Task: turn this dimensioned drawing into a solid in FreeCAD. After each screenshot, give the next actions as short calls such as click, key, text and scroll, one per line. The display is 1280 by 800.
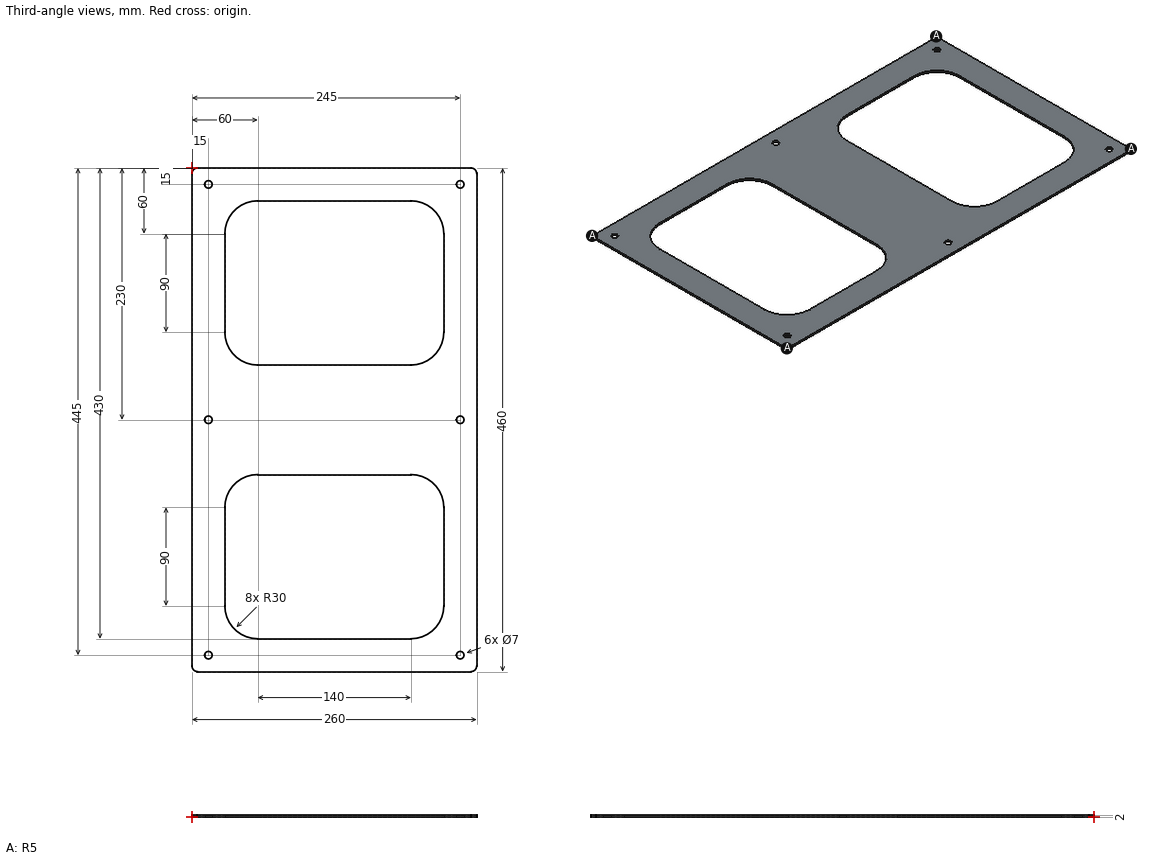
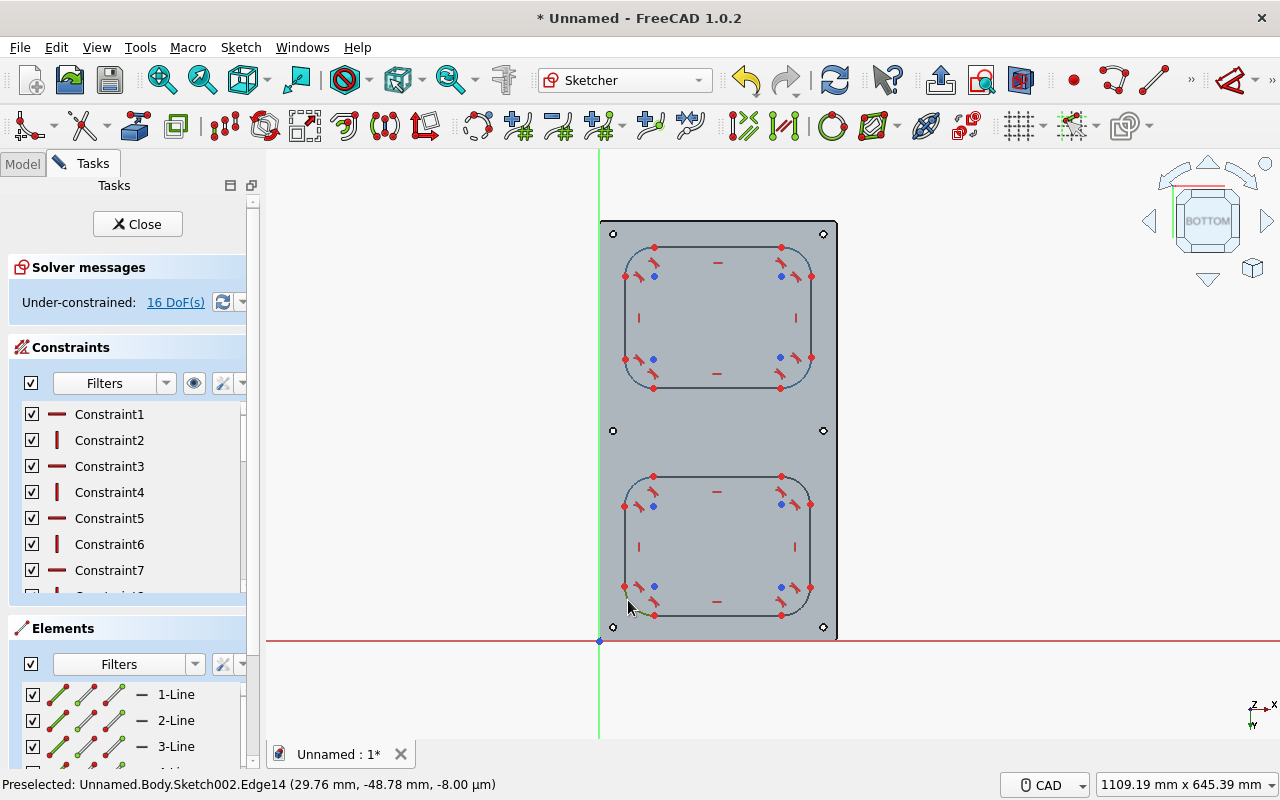
click(794, 613)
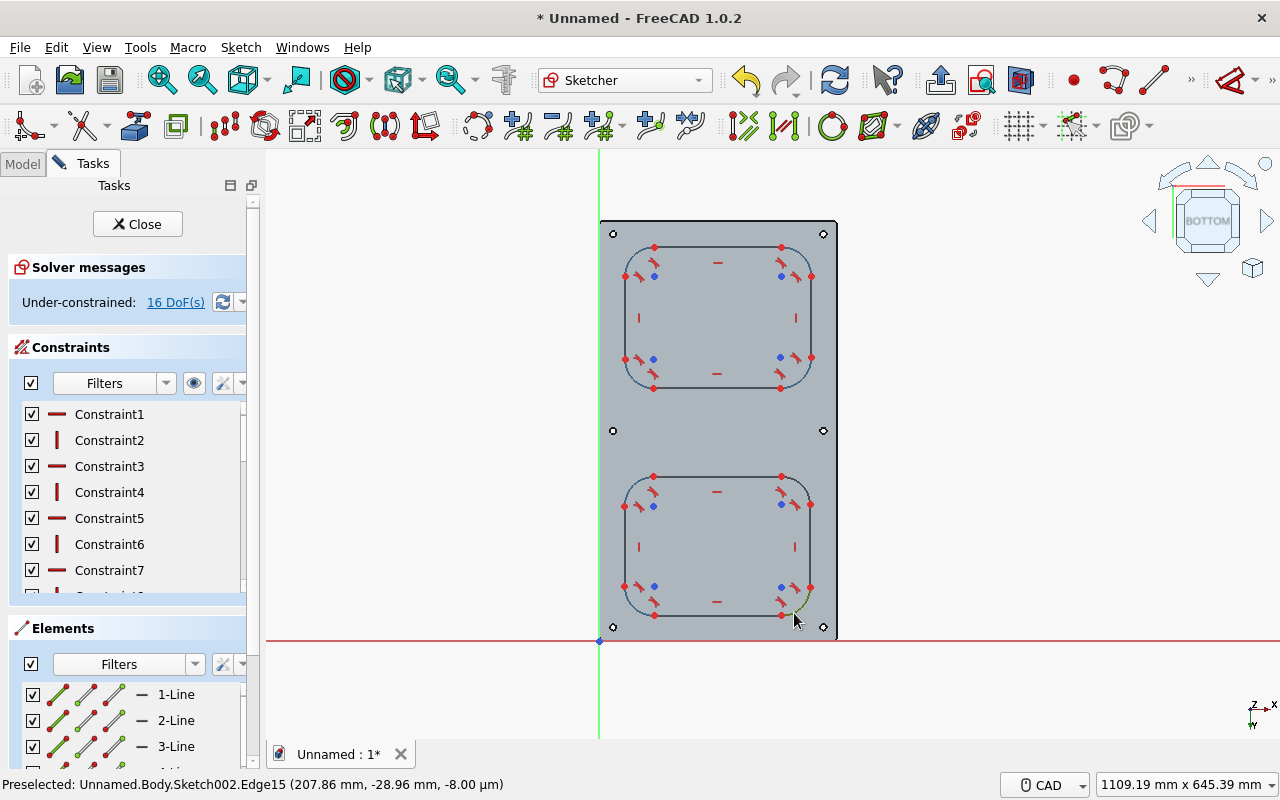
click(807, 492)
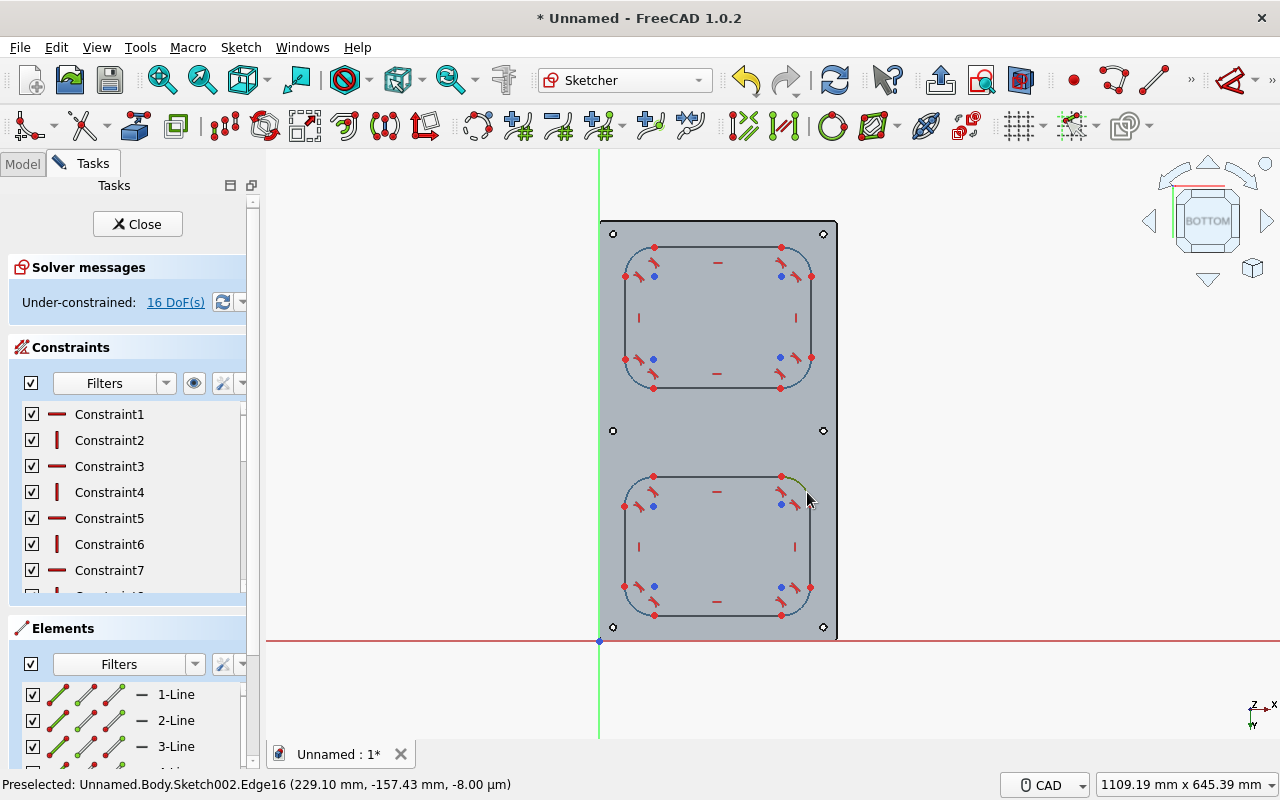
key(e)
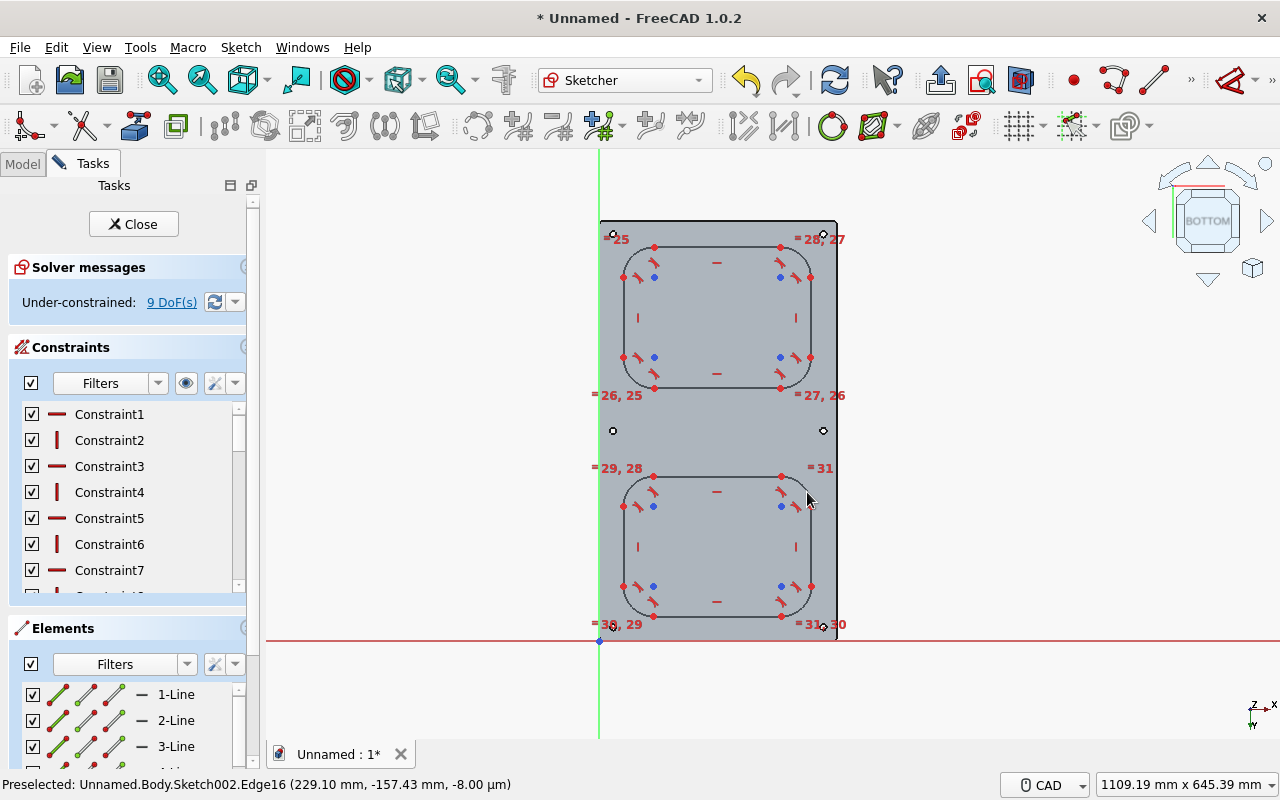
click(1230, 80)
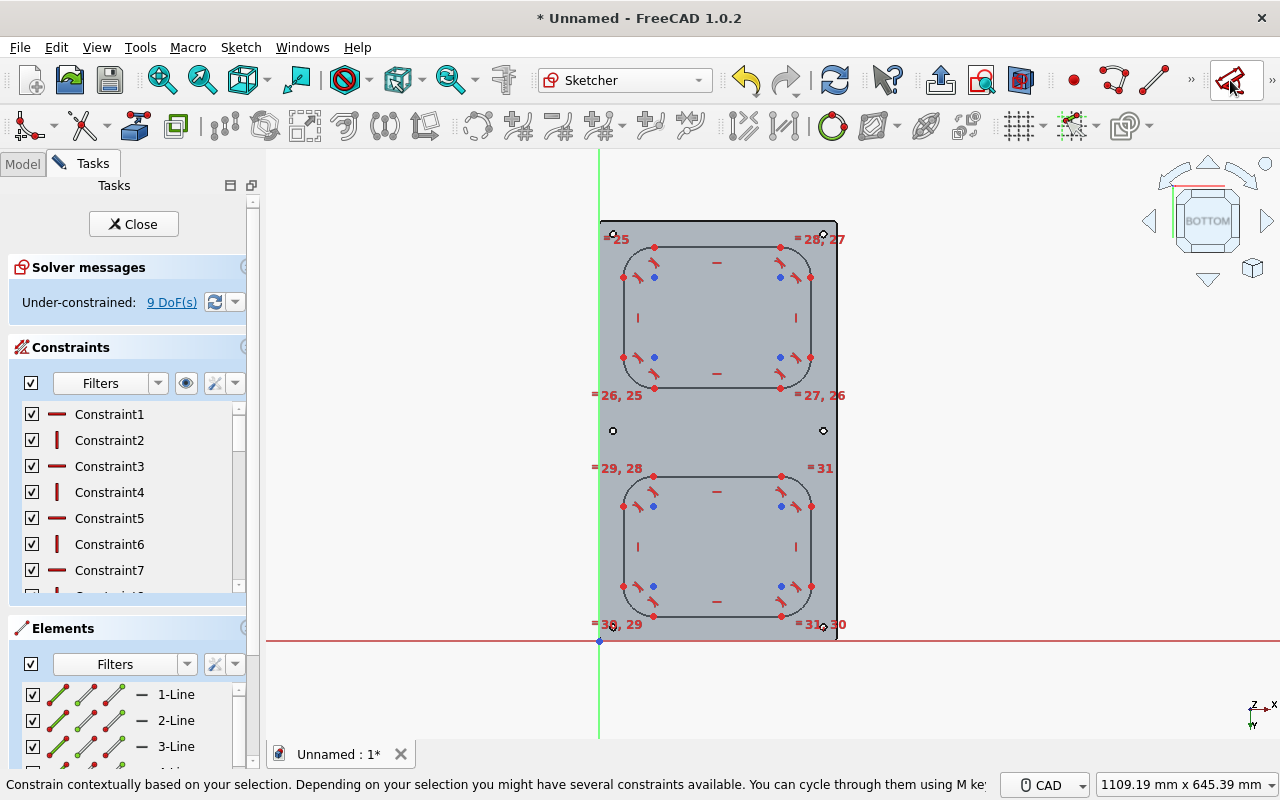
scroll(640, 251, up, 2)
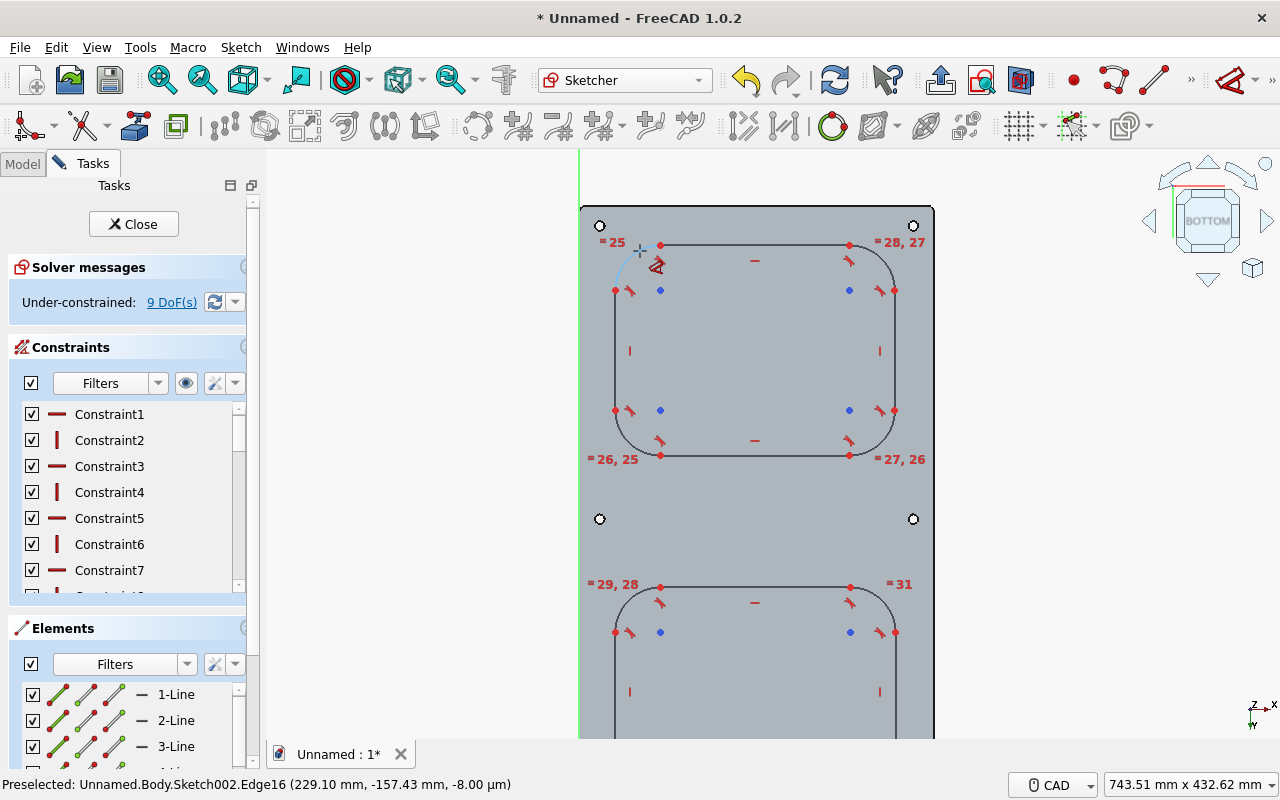
click(640, 250)
click(626, 221)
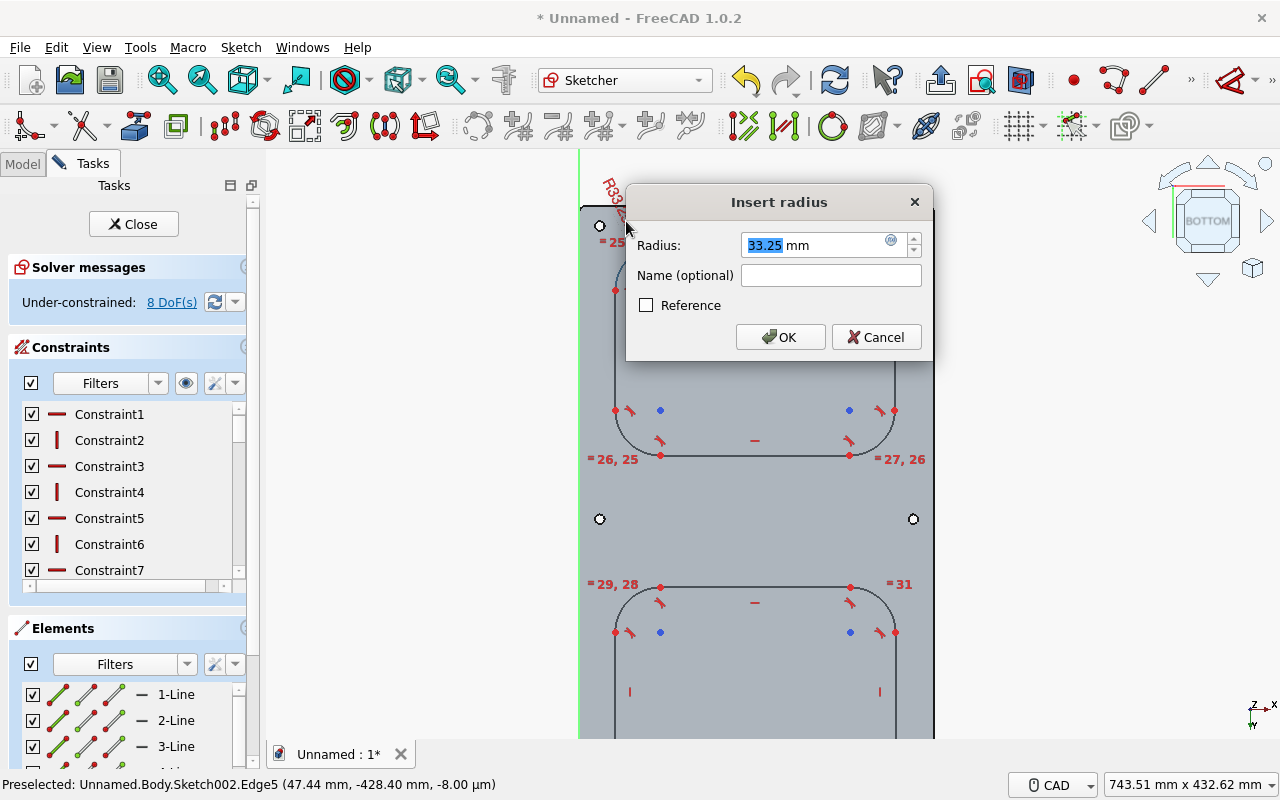
text(30)
key(Return)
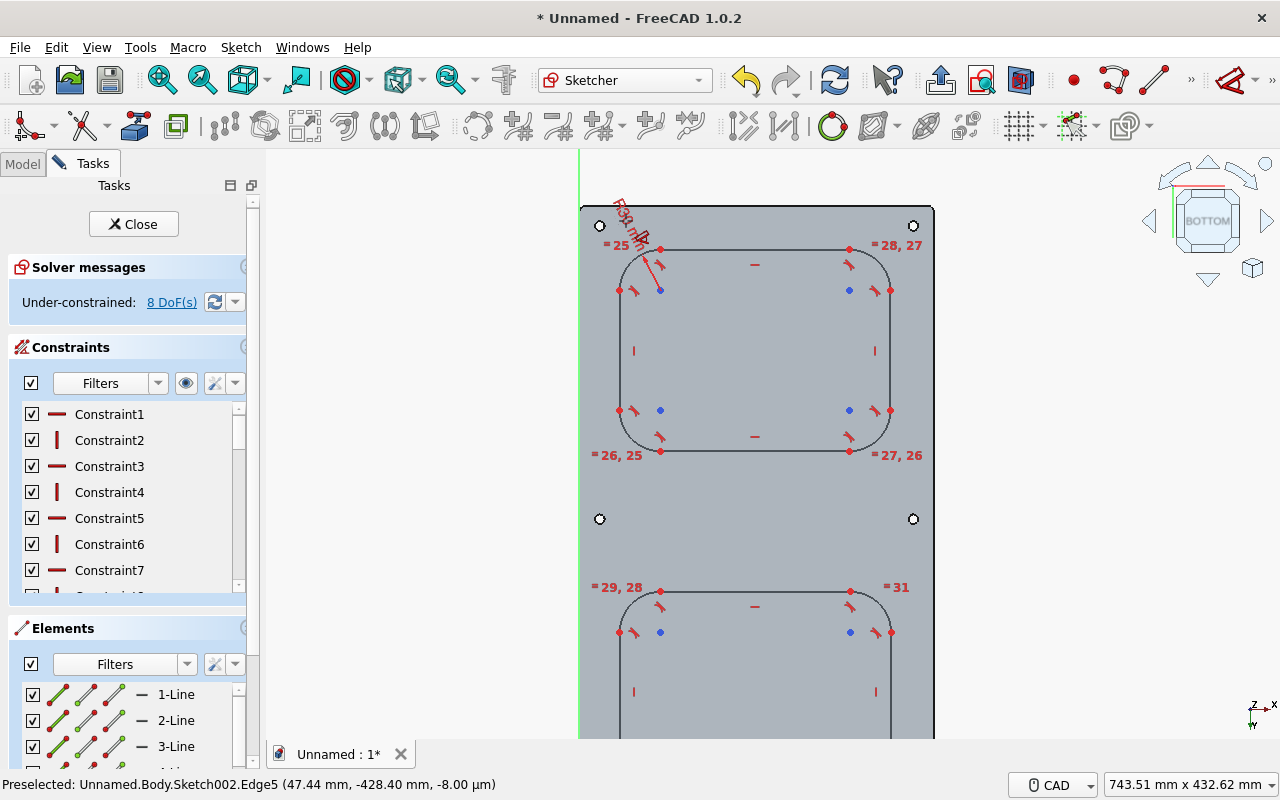
click(620, 327)
click(654, 351)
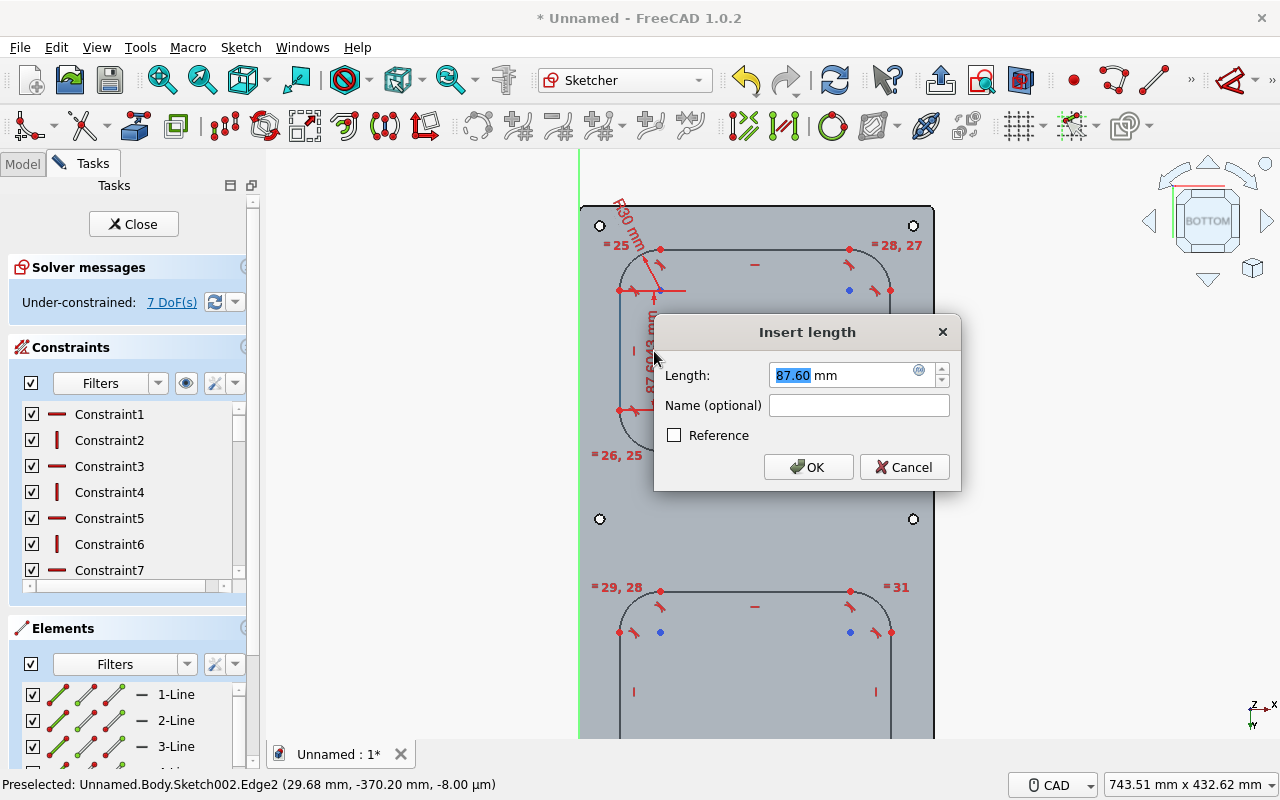
text(90)
key(Return)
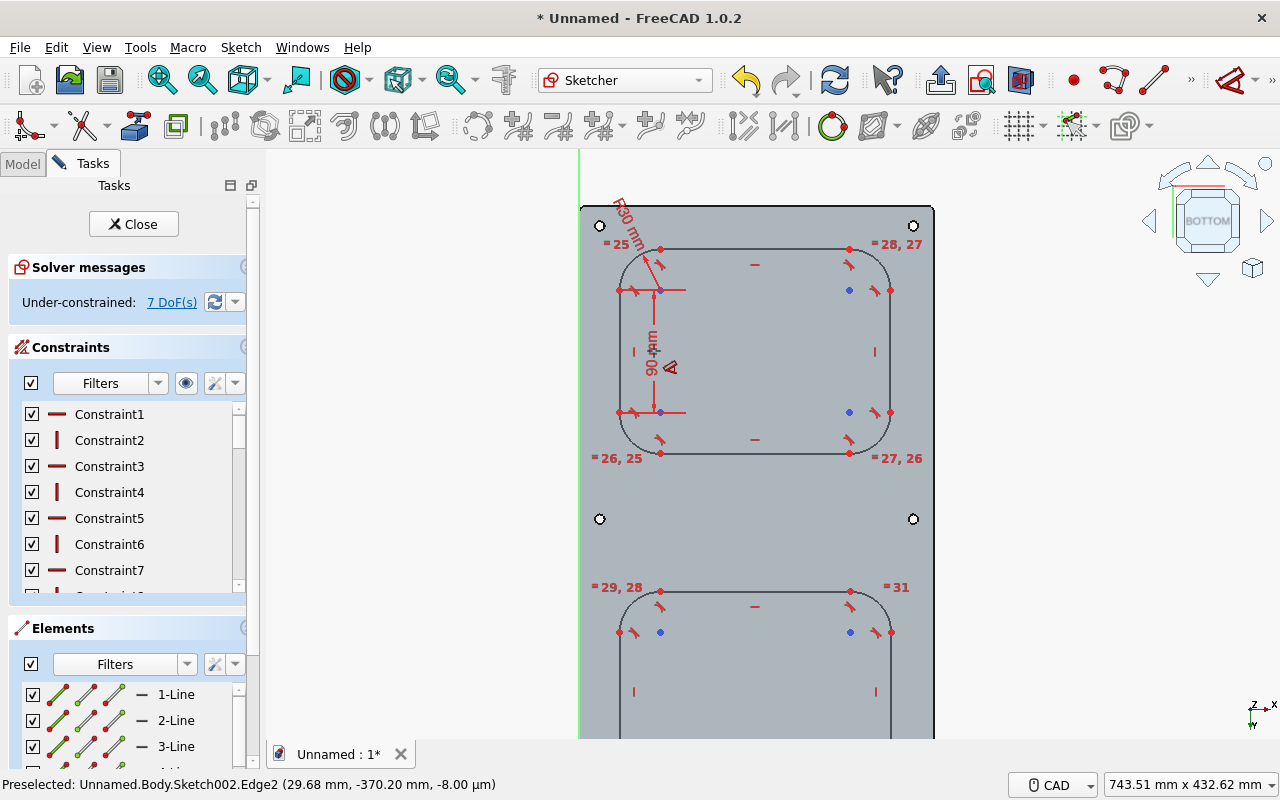
click(620, 668)
click(654, 672)